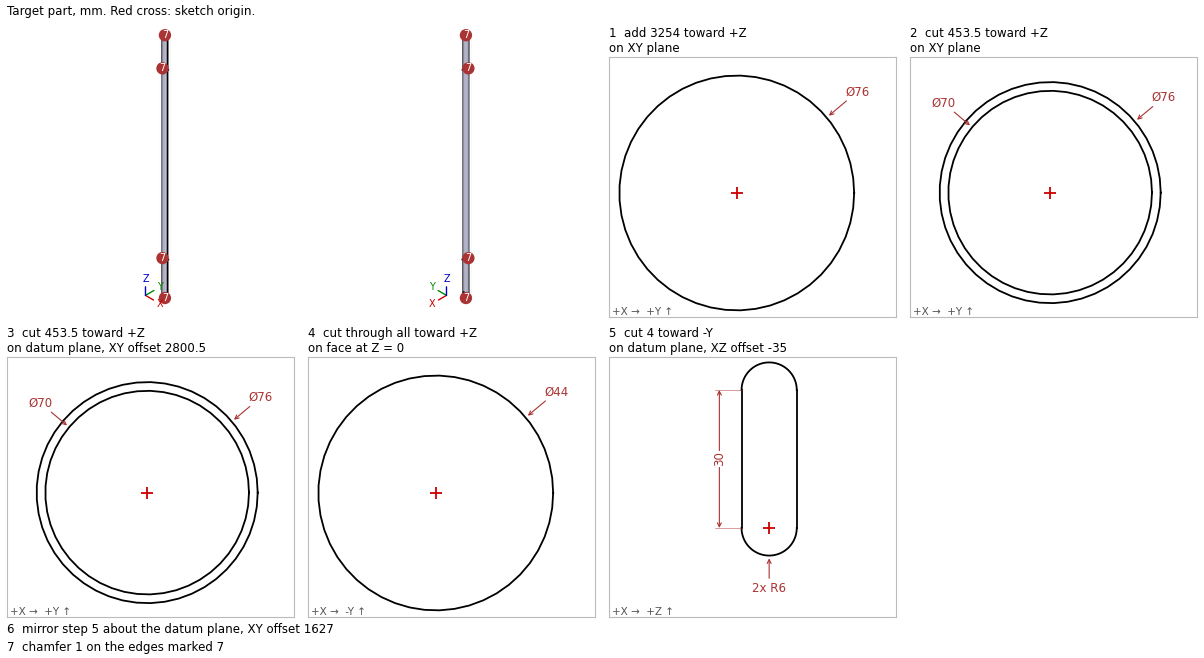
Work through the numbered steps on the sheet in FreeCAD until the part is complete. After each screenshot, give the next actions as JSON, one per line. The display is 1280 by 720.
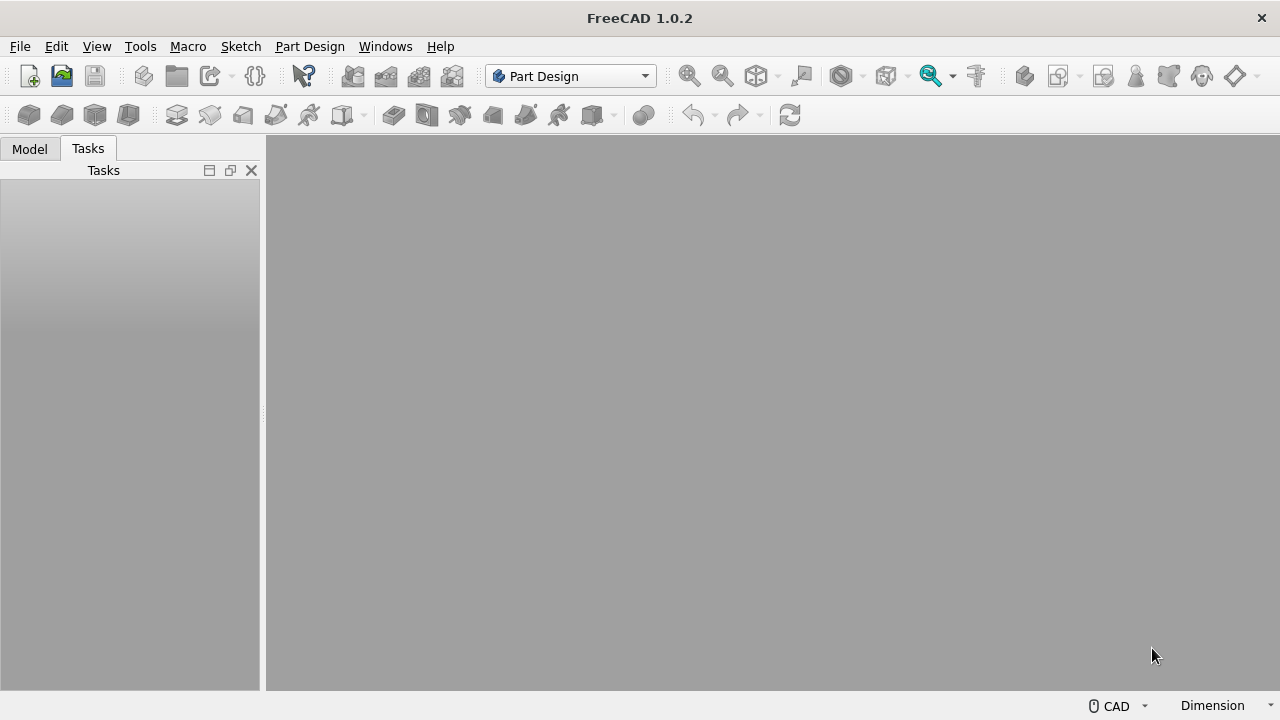
{"action": "left_click", "coordinate": [29, 76]}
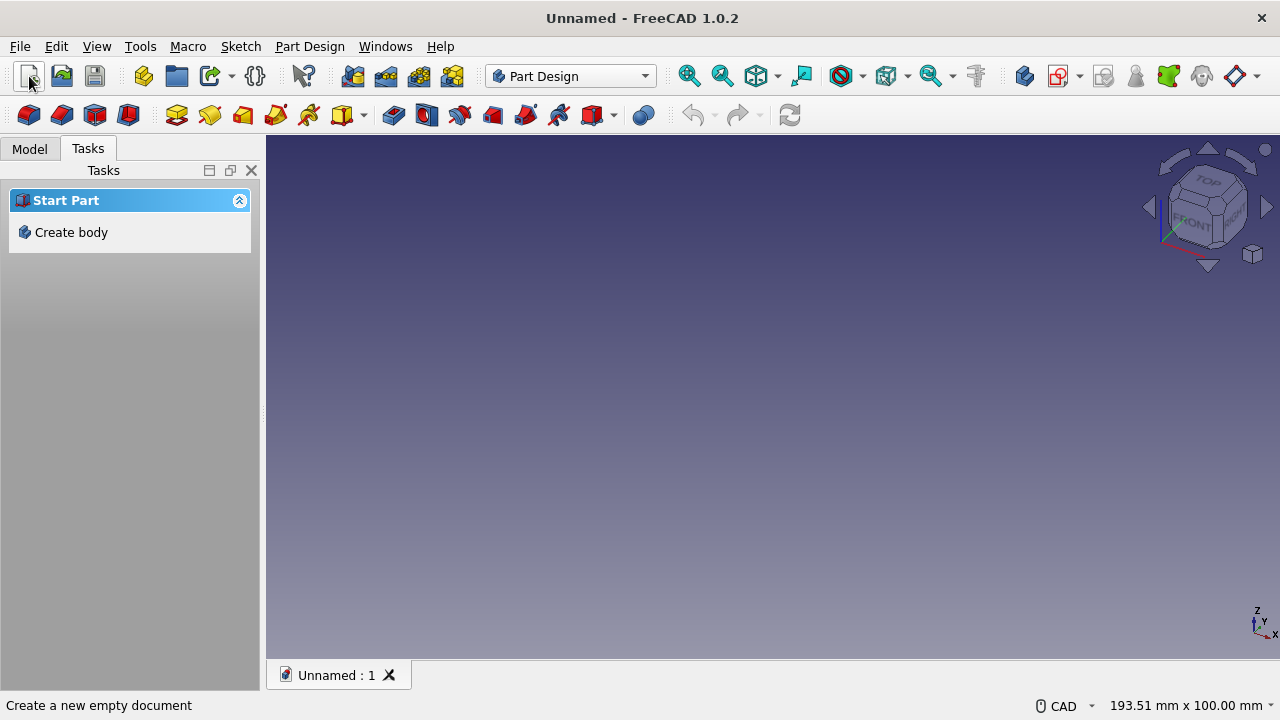
{"action": "left_click", "coordinate": [1058, 76]}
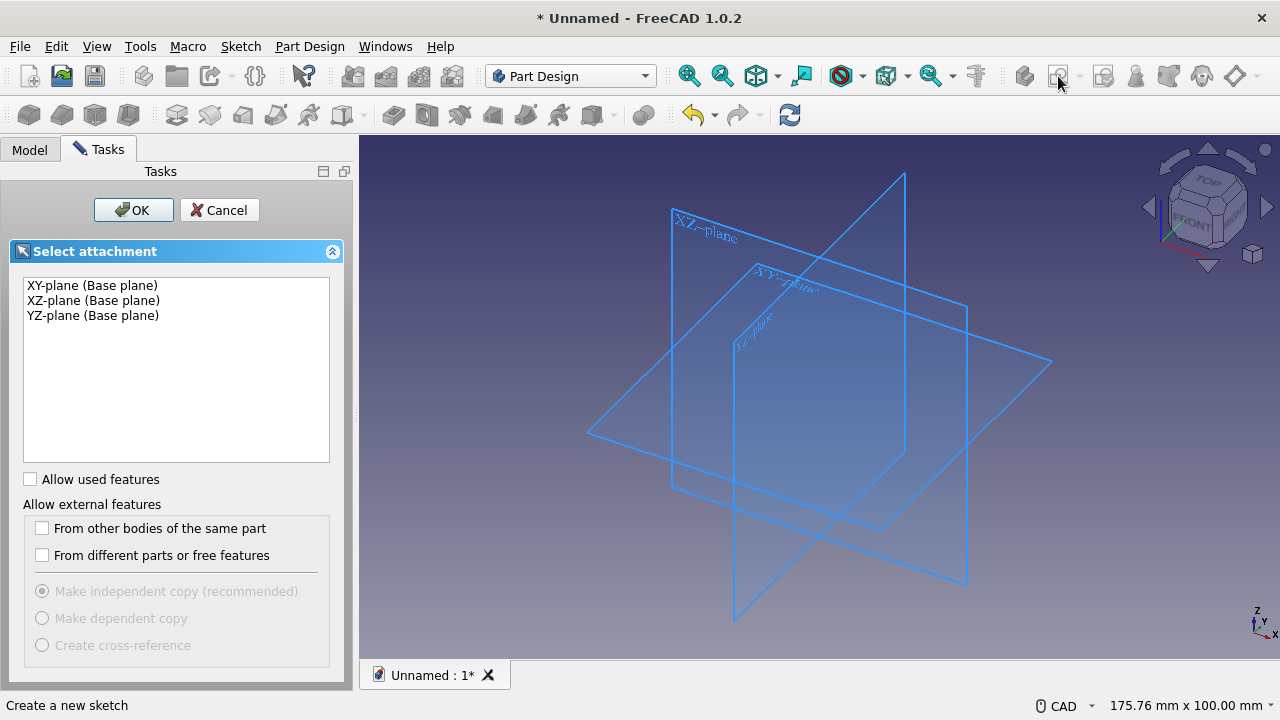
{"action": "left_click", "coordinate": [84, 286]}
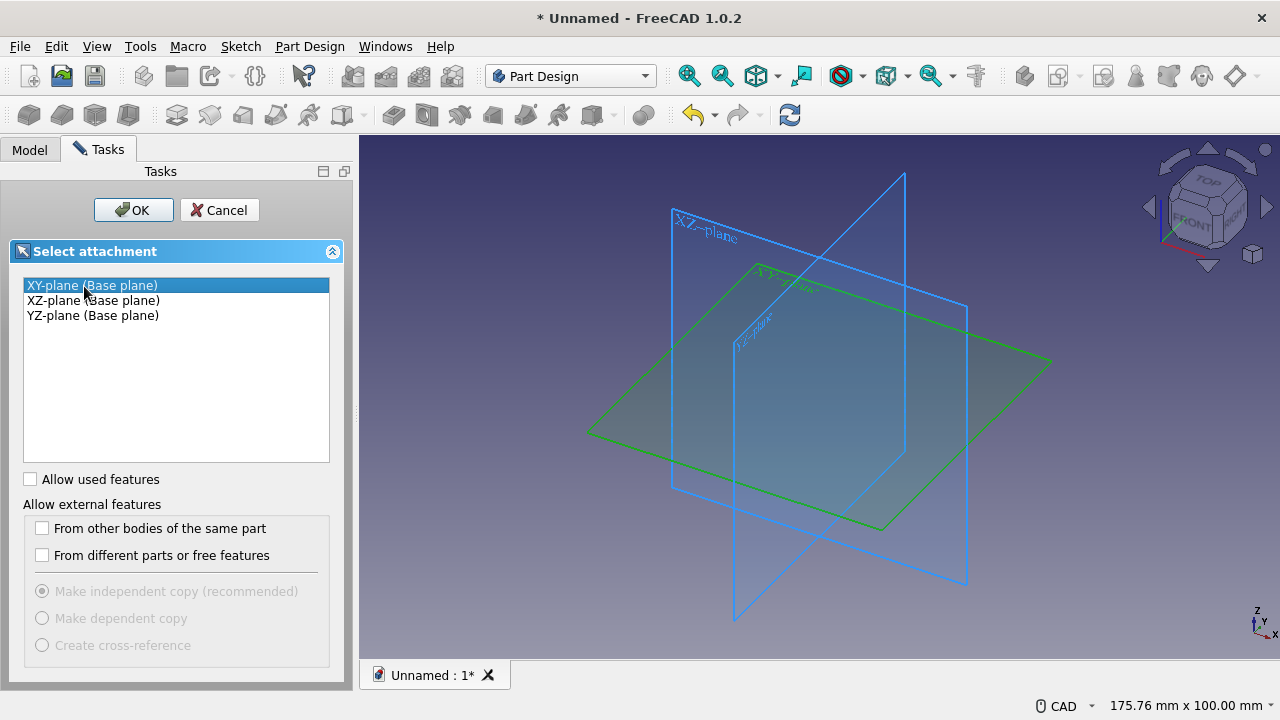
{"action": "left_click", "coordinate": [134, 210]}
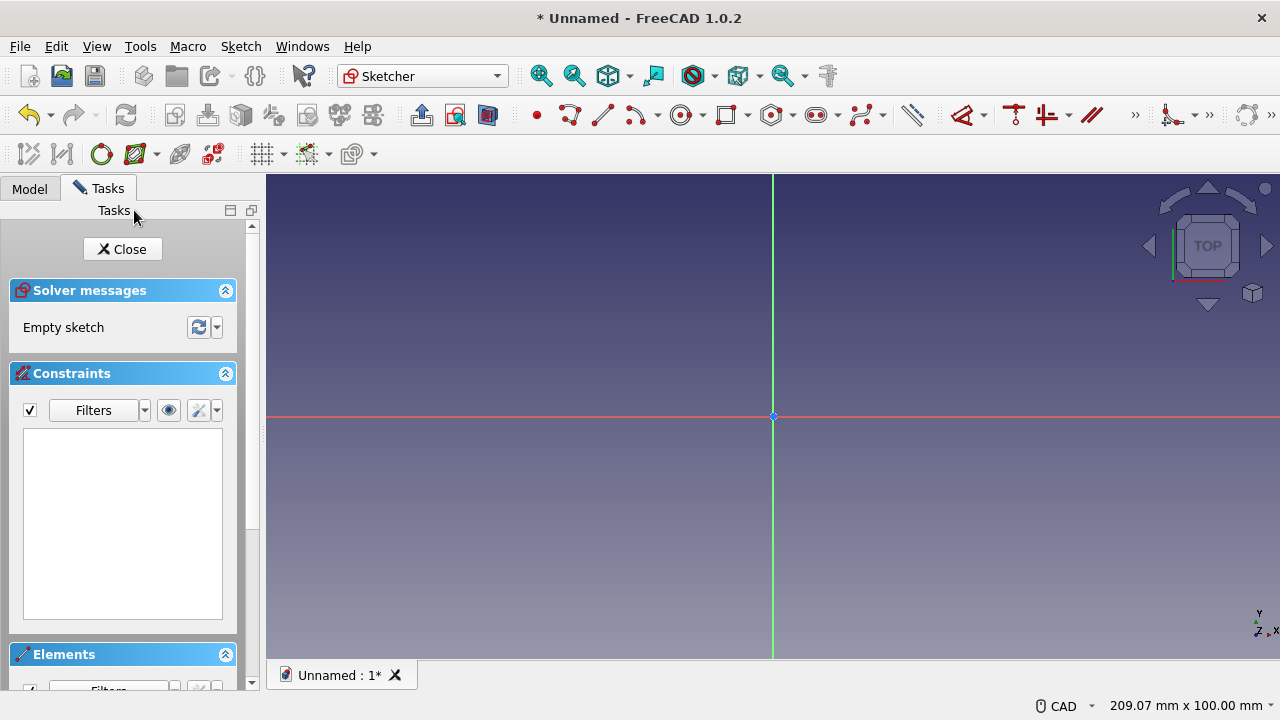
{"action": "left_click", "coordinate": [680, 116]}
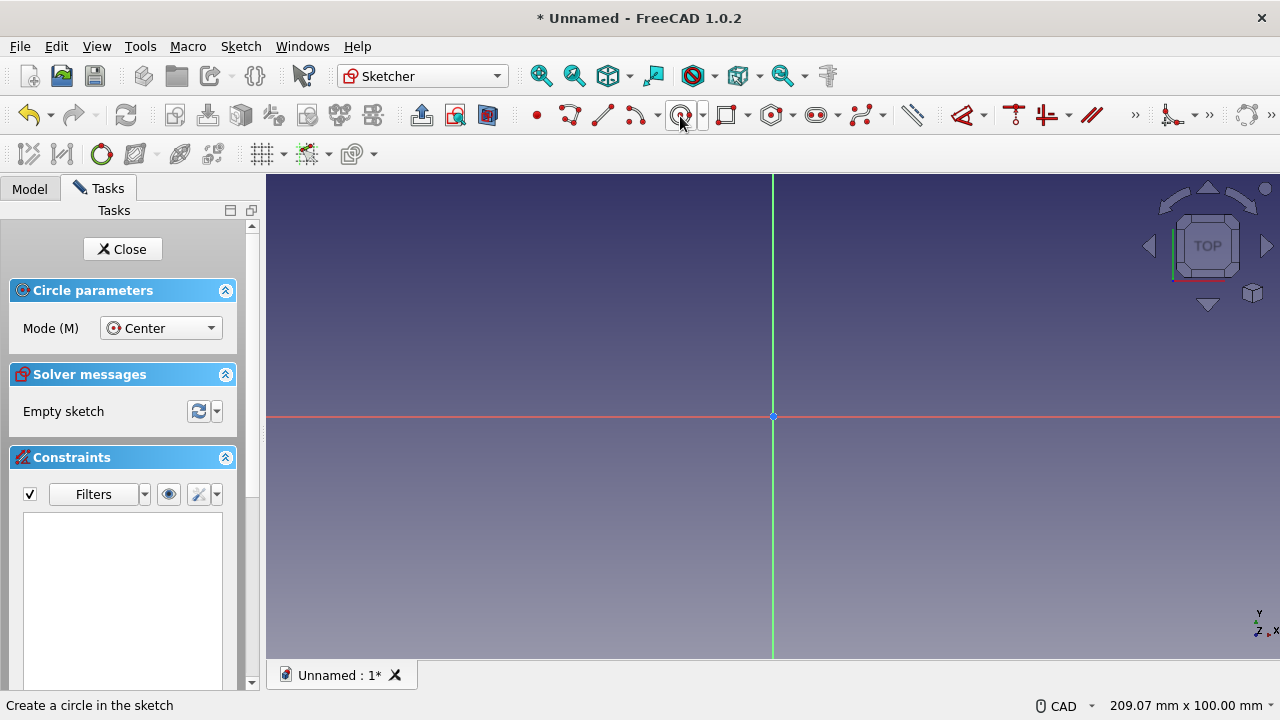
{"action": "left_click", "coordinate": [773, 416]}
{"action": "left_click", "coordinate": [903, 286]}
{"action": "key", "text": "Escape"}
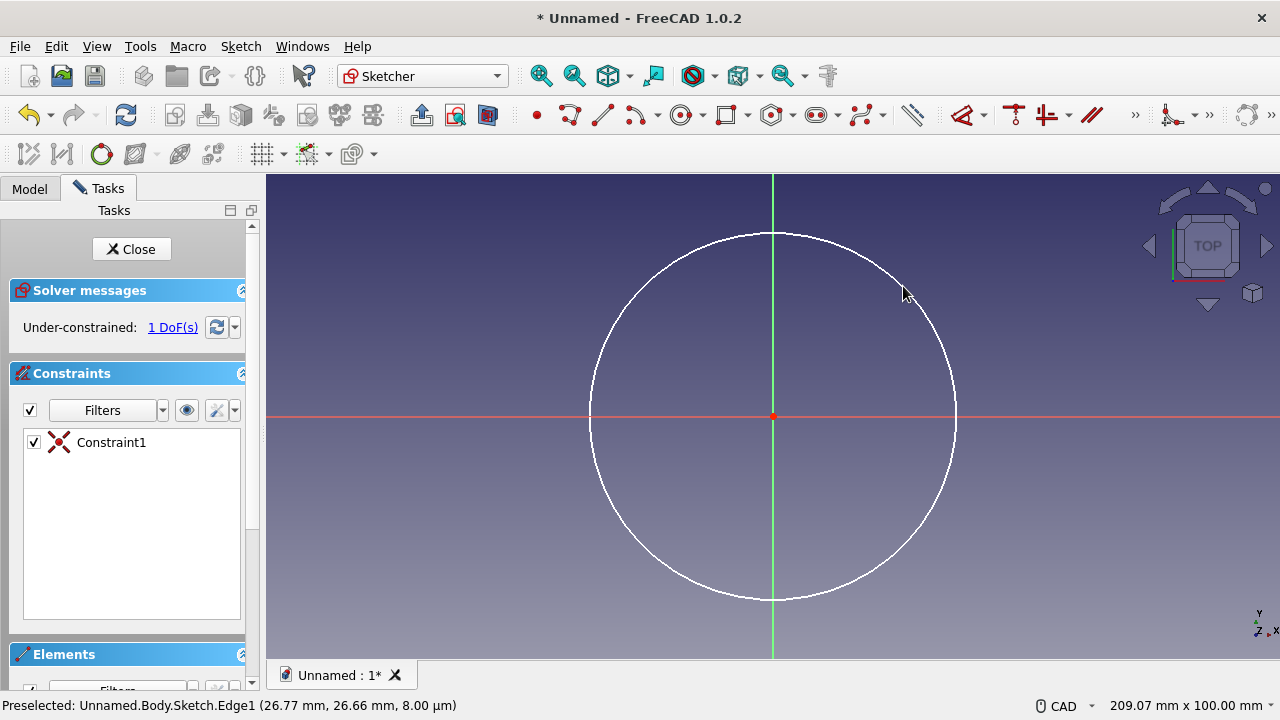
{"action": "left_click", "coordinate": [902, 286]}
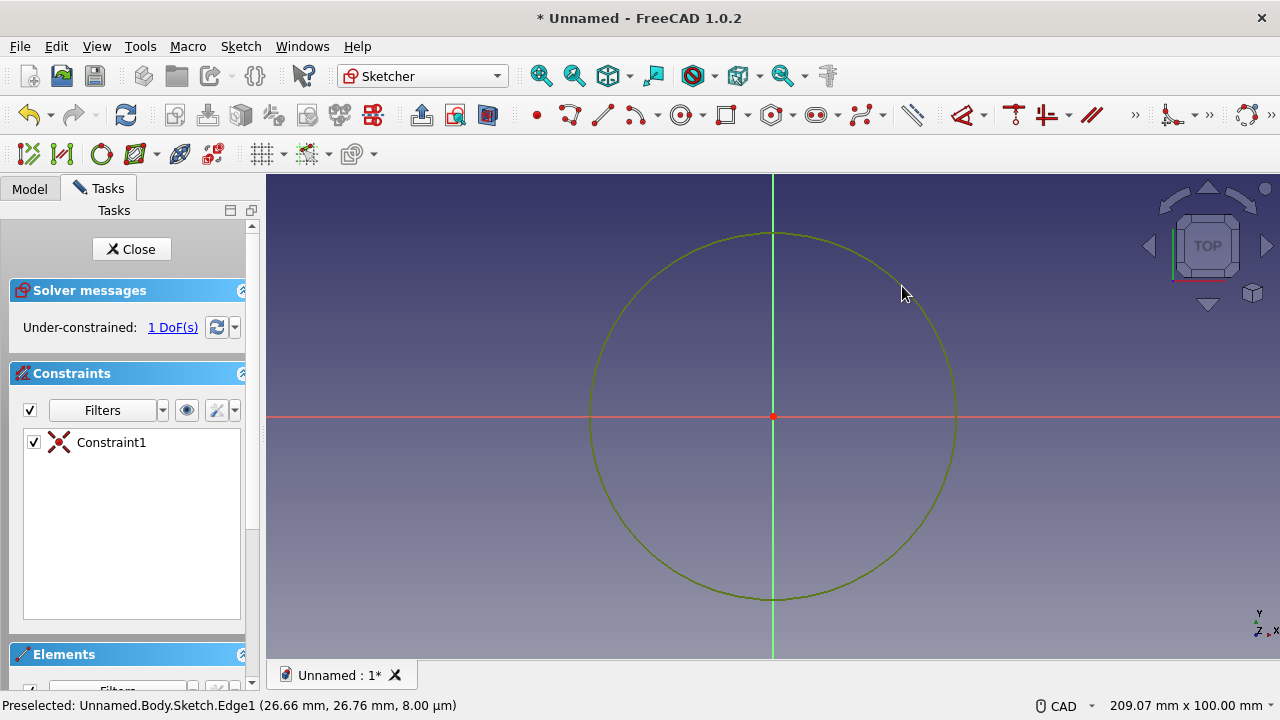
{"action": "key", "text": "k o"}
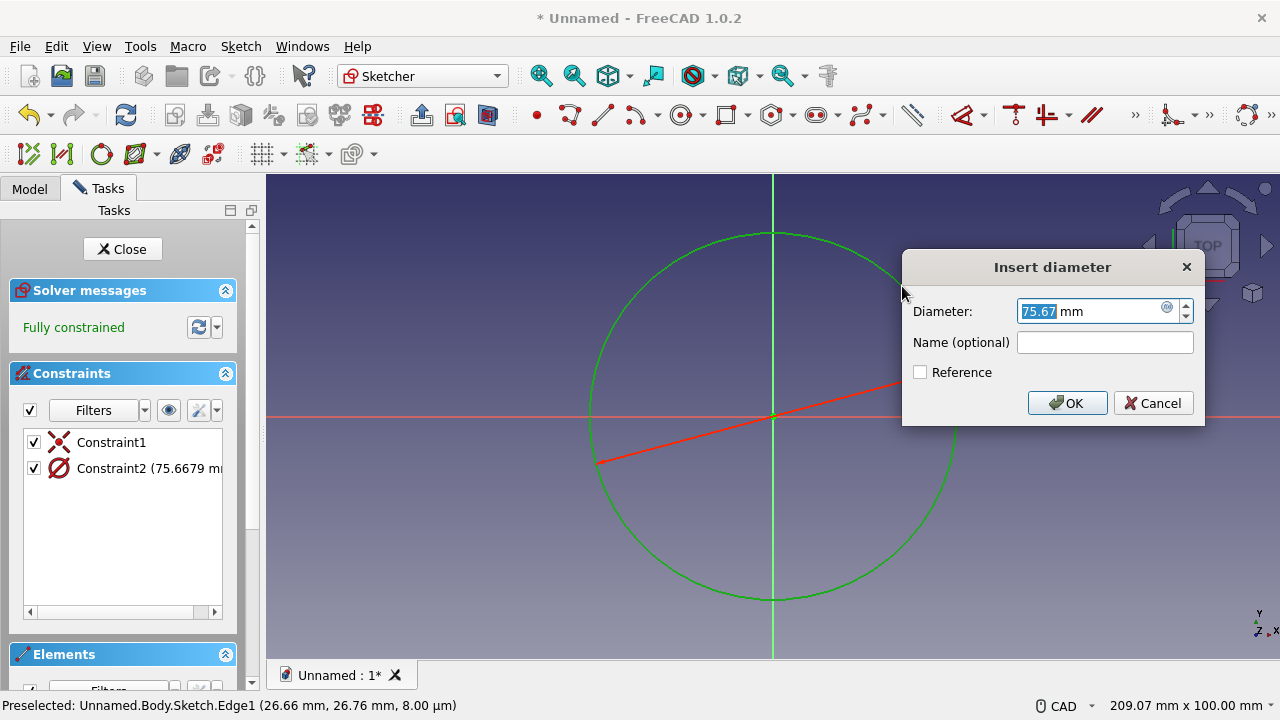
{"action": "type", "text": "76"}
{"action": "key", "text": "Return"}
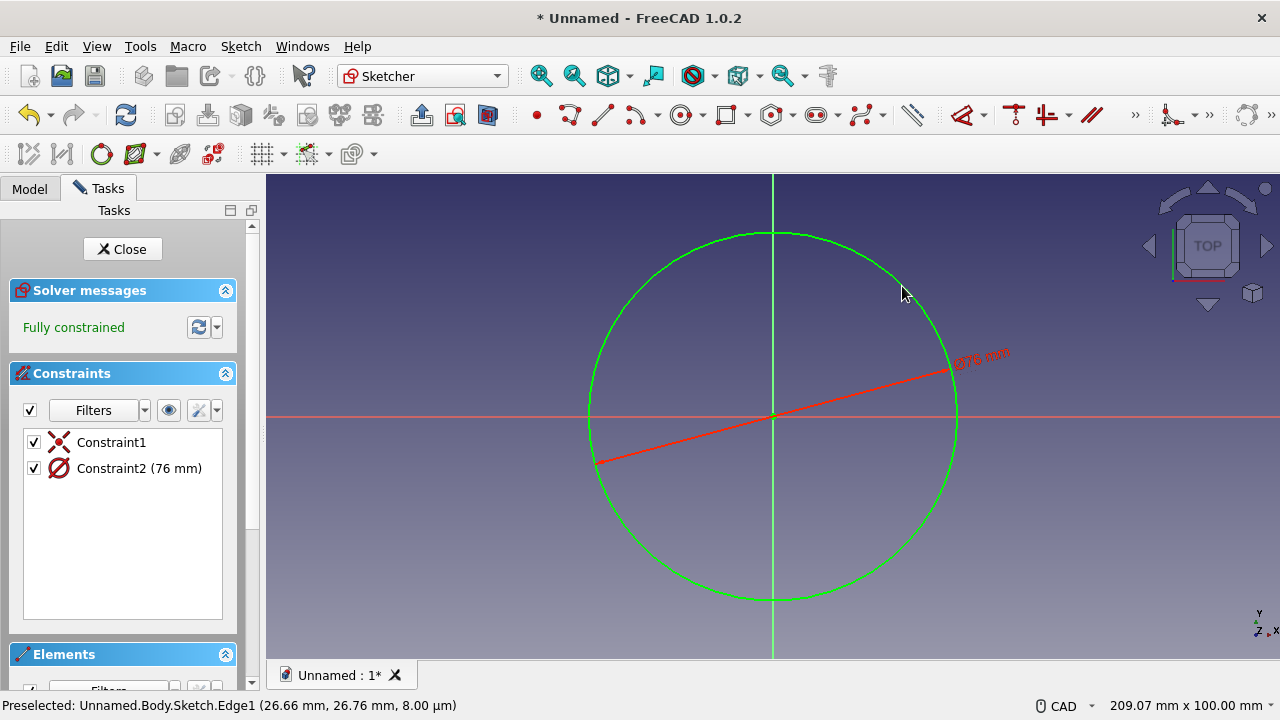
{"action": "left_click", "coordinate": [123, 249]}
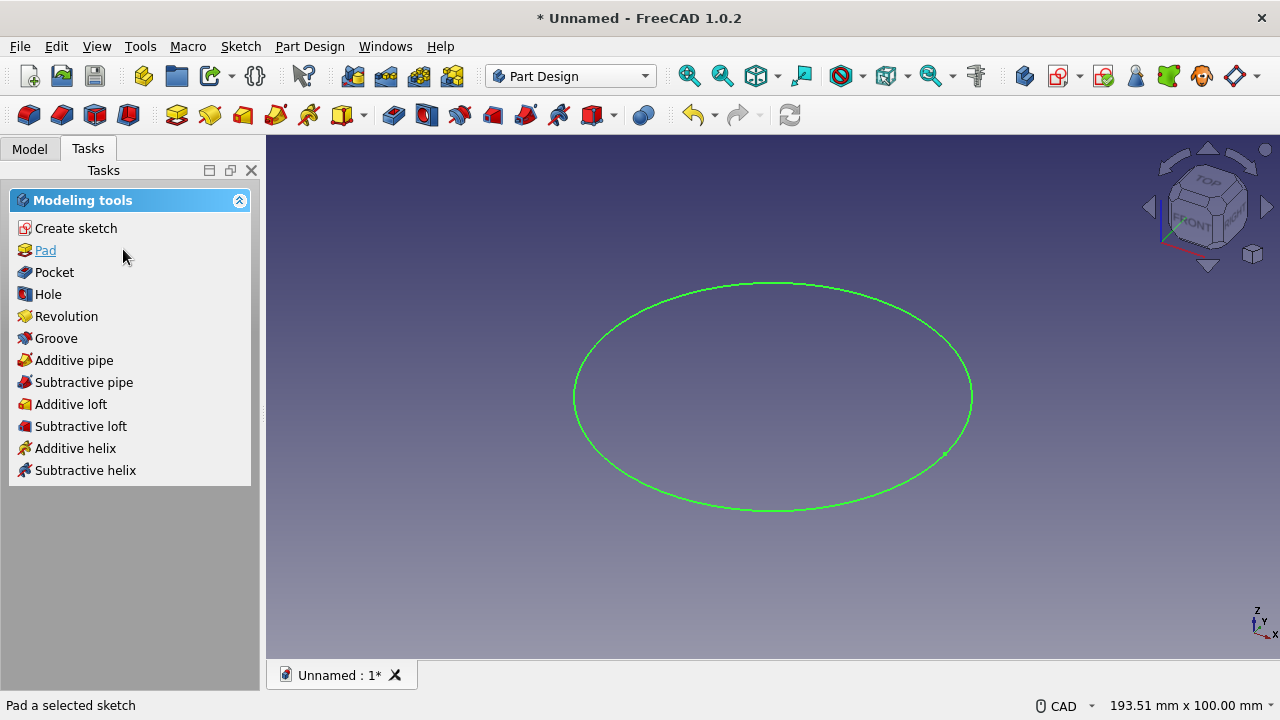
{"action": "left_click", "coordinate": [177, 116]}